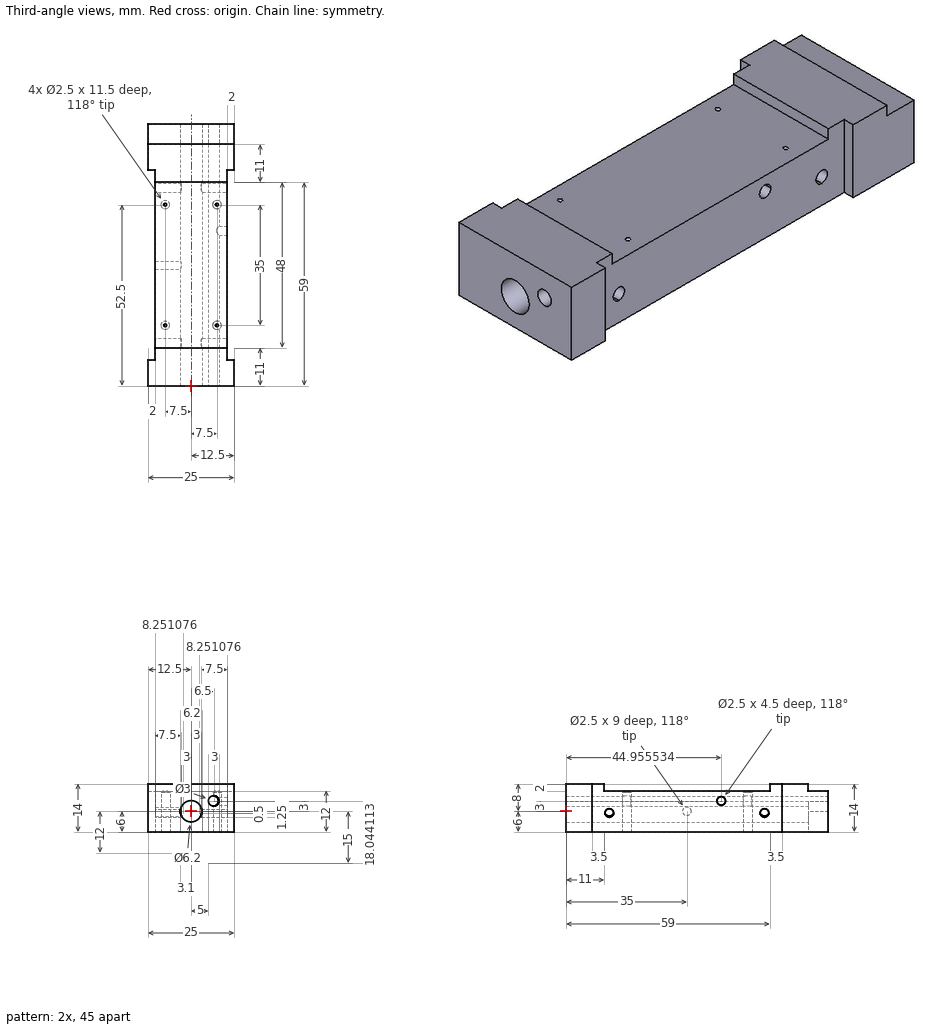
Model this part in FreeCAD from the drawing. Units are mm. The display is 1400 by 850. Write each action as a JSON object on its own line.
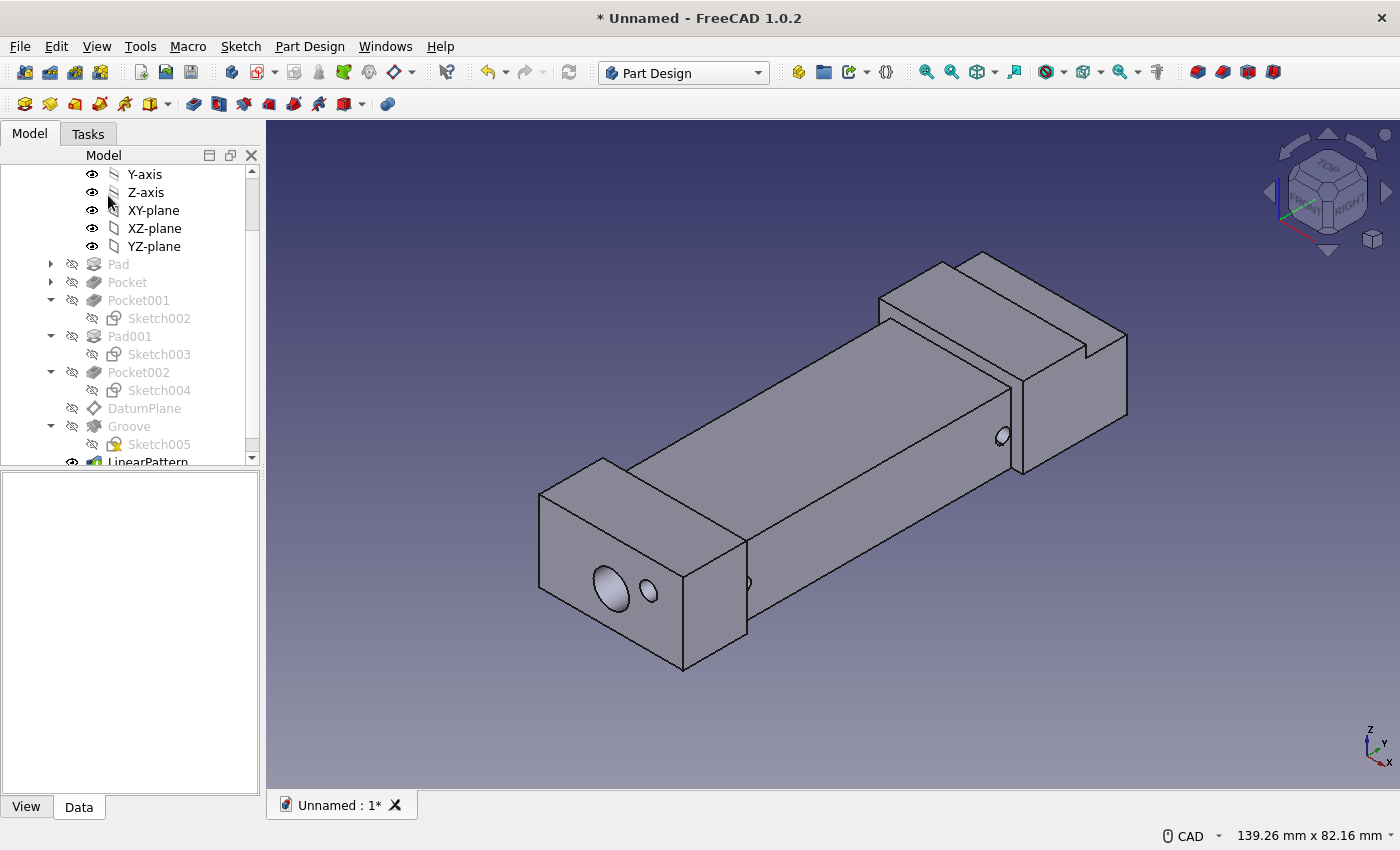
{"action": "left_click", "coordinate": [117, 426]}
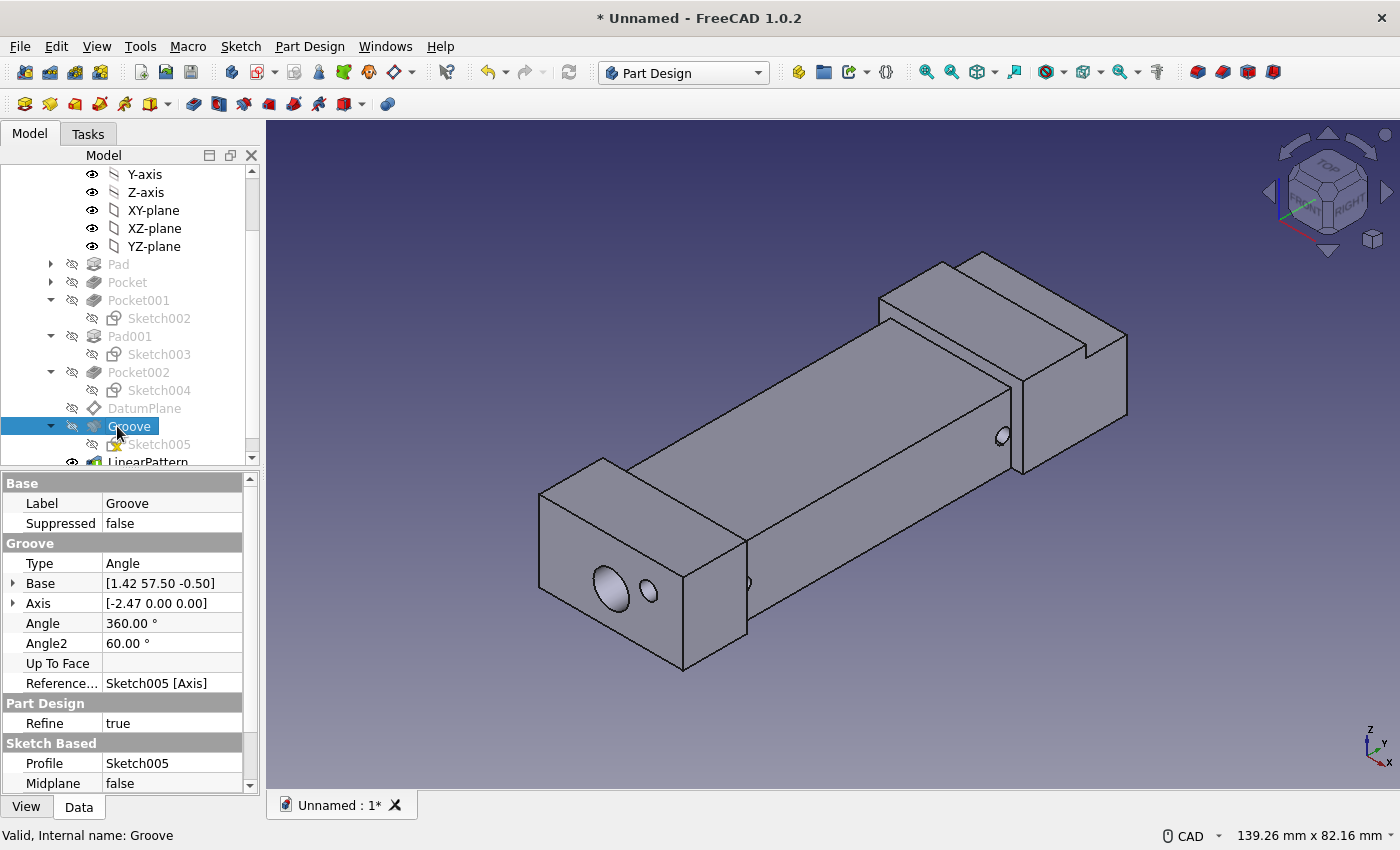
{"action": "left_click", "coordinate": [25, 72]}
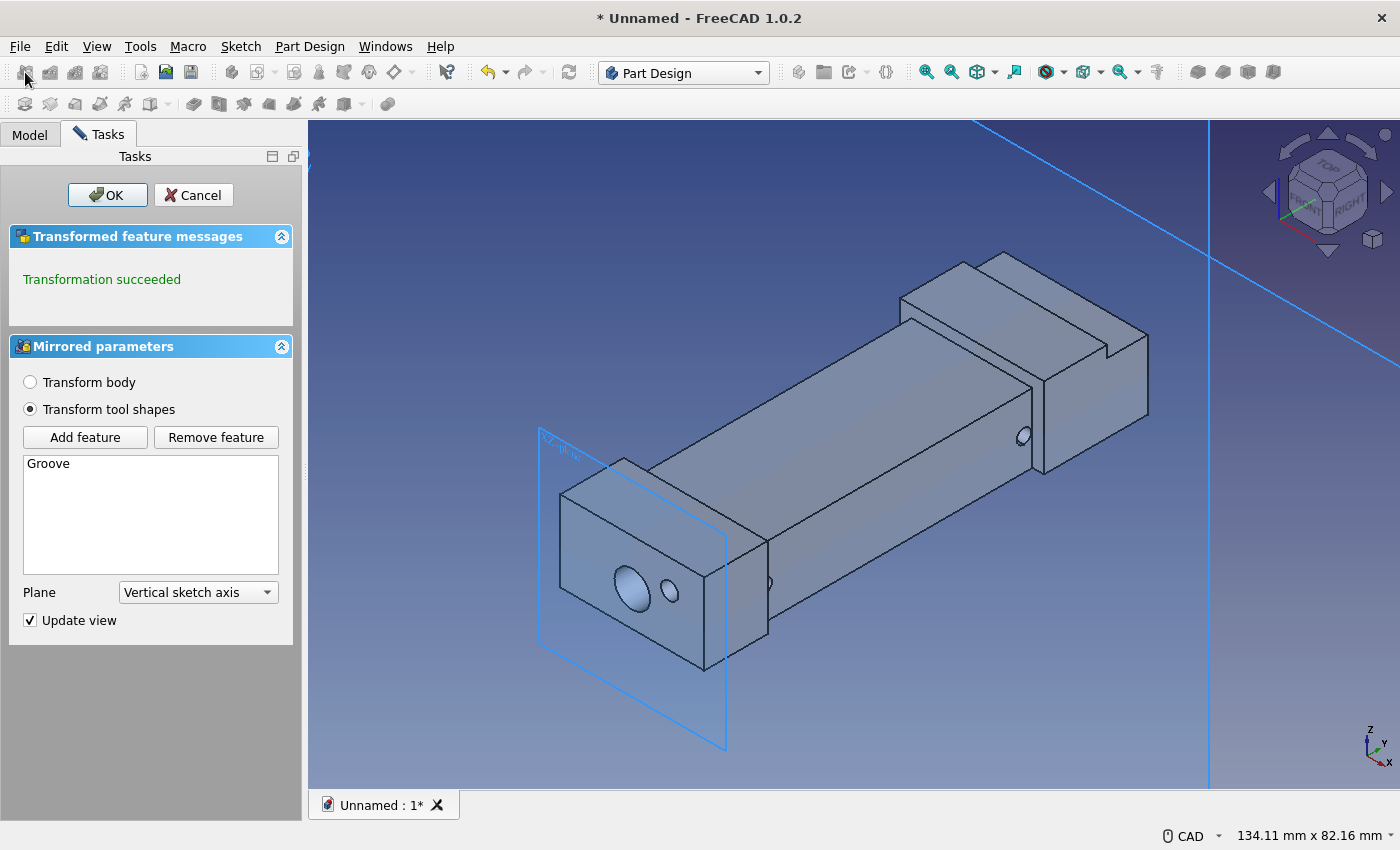
{"action": "left_click", "coordinate": [199, 592]}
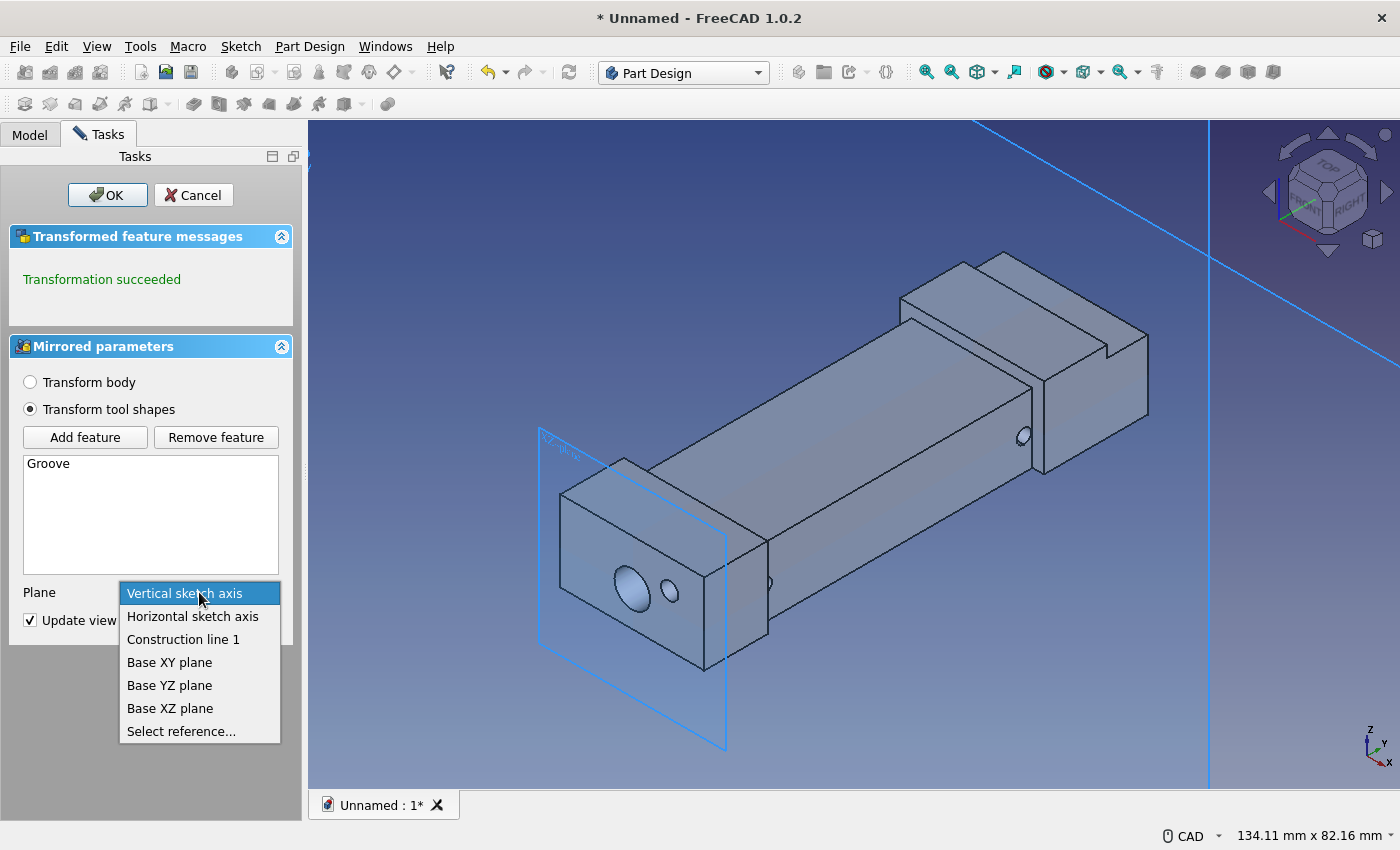
{"action": "left_click", "coordinate": [198, 686]}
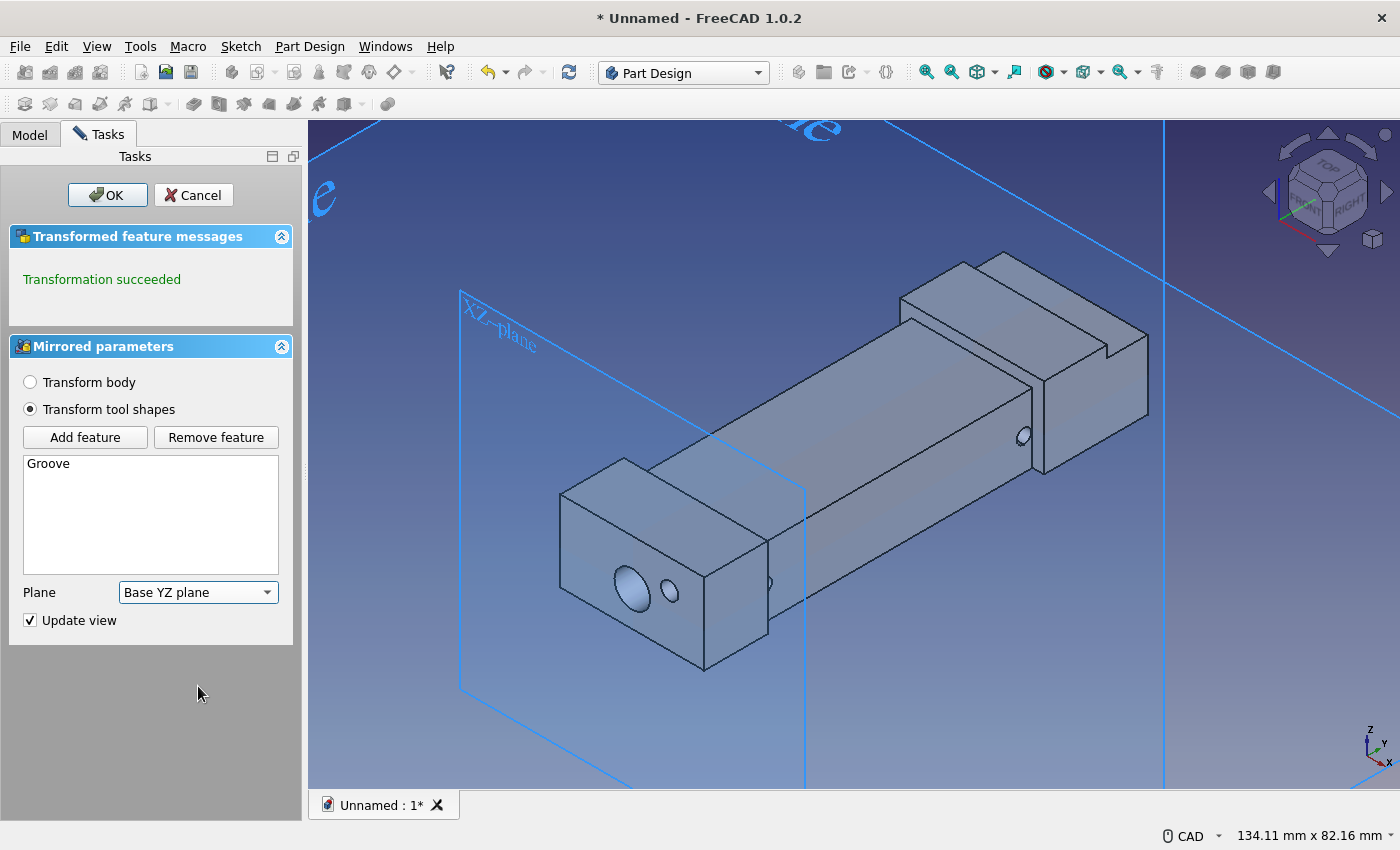
{"action": "left_click", "coordinate": [108, 195]}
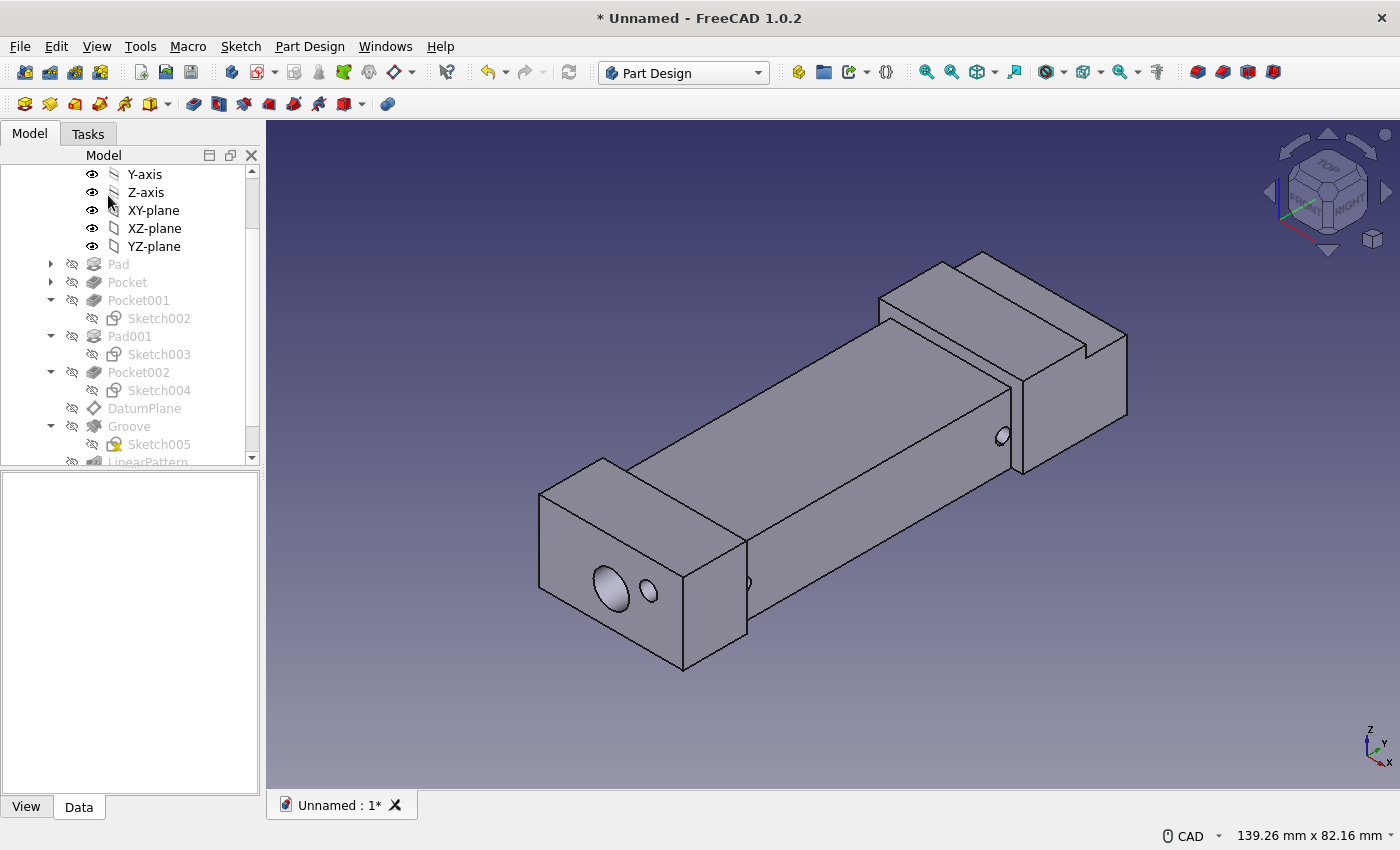
{"action": "scroll", "coordinate": [161, 314], "scroll_direction": "down", "scroll_amount": 3}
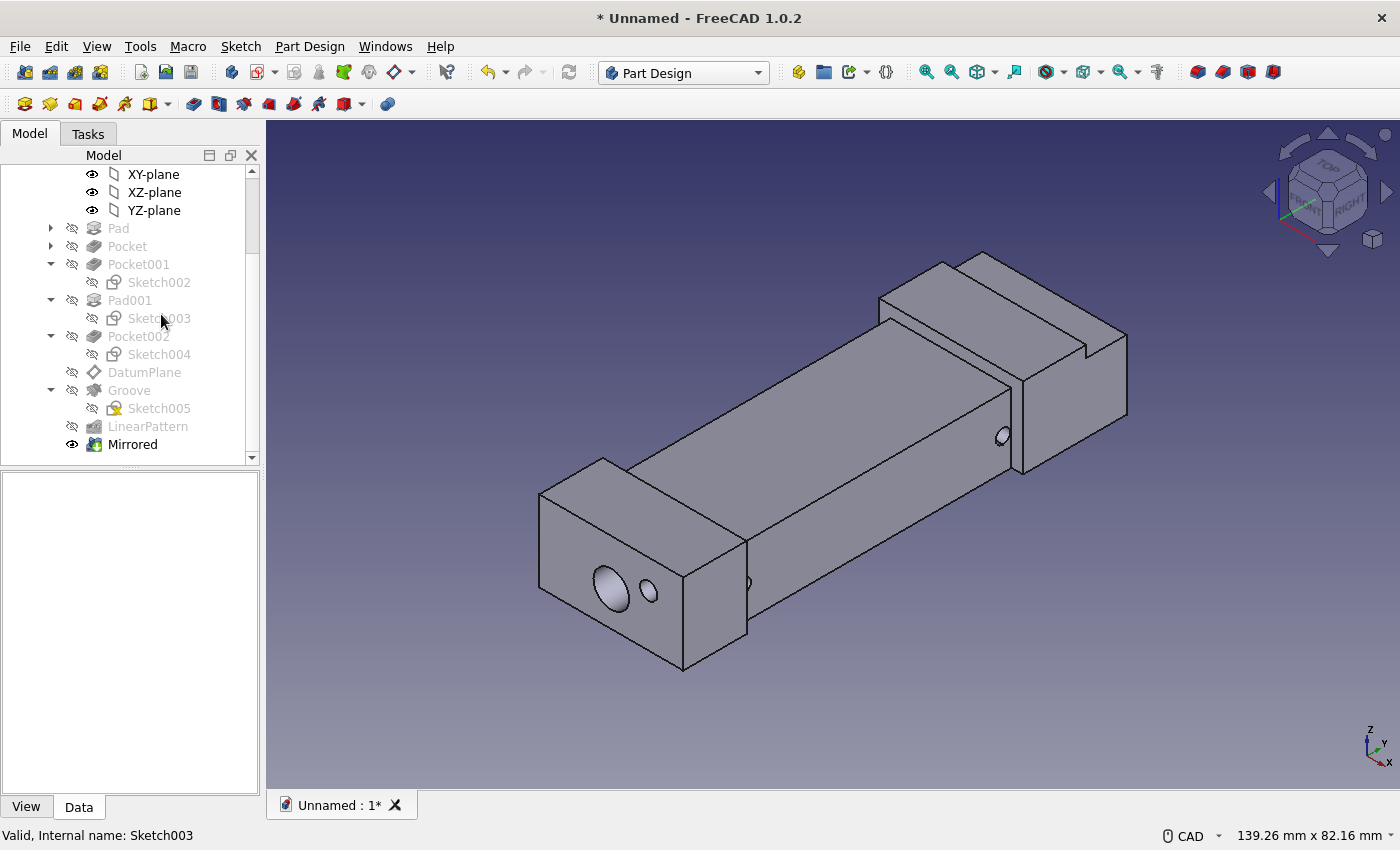
{"action": "scroll", "coordinate": [161, 314], "scroll_direction": "up", "scroll_amount": 15}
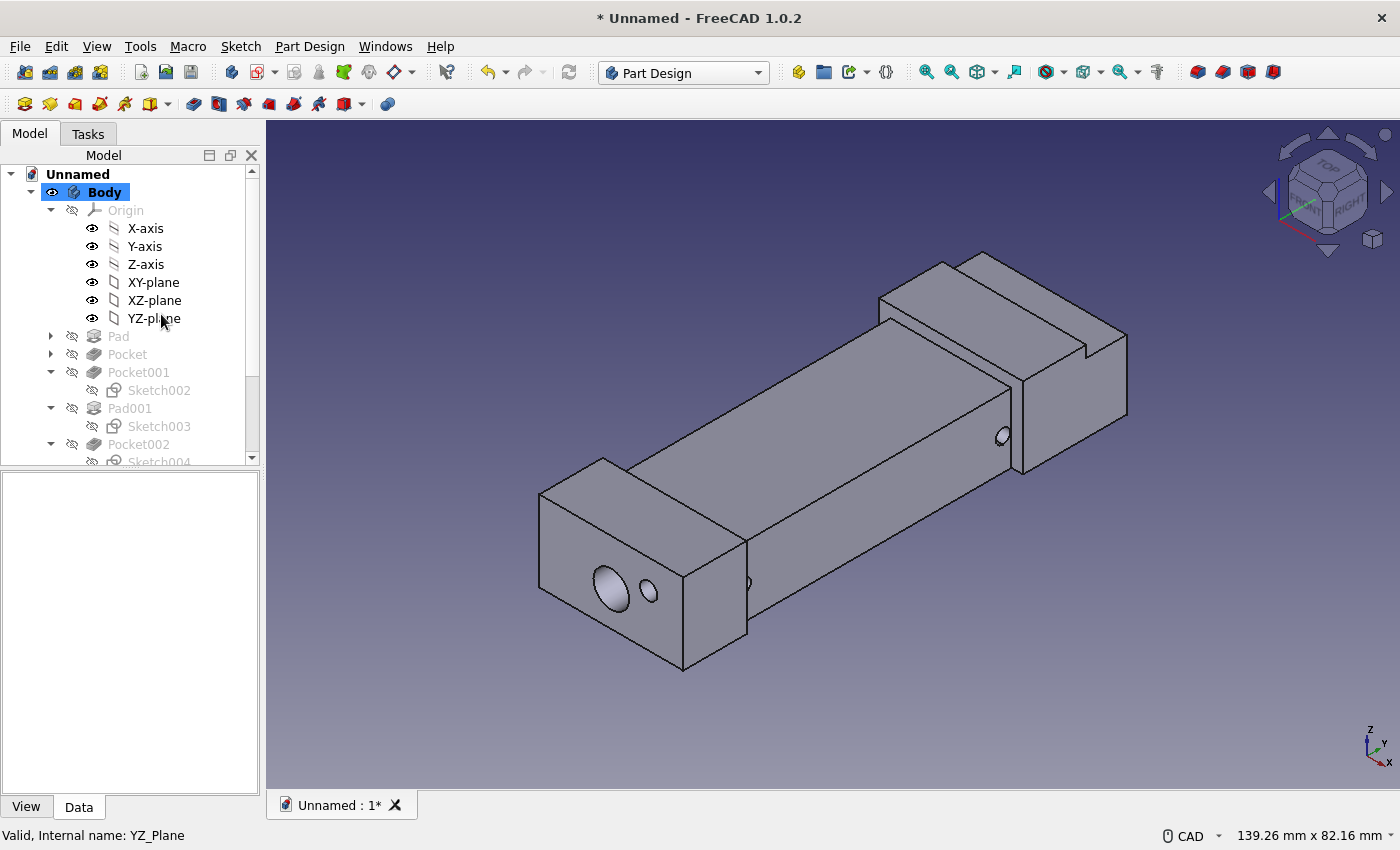
{"action": "left_click", "coordinate": [137, 300]}